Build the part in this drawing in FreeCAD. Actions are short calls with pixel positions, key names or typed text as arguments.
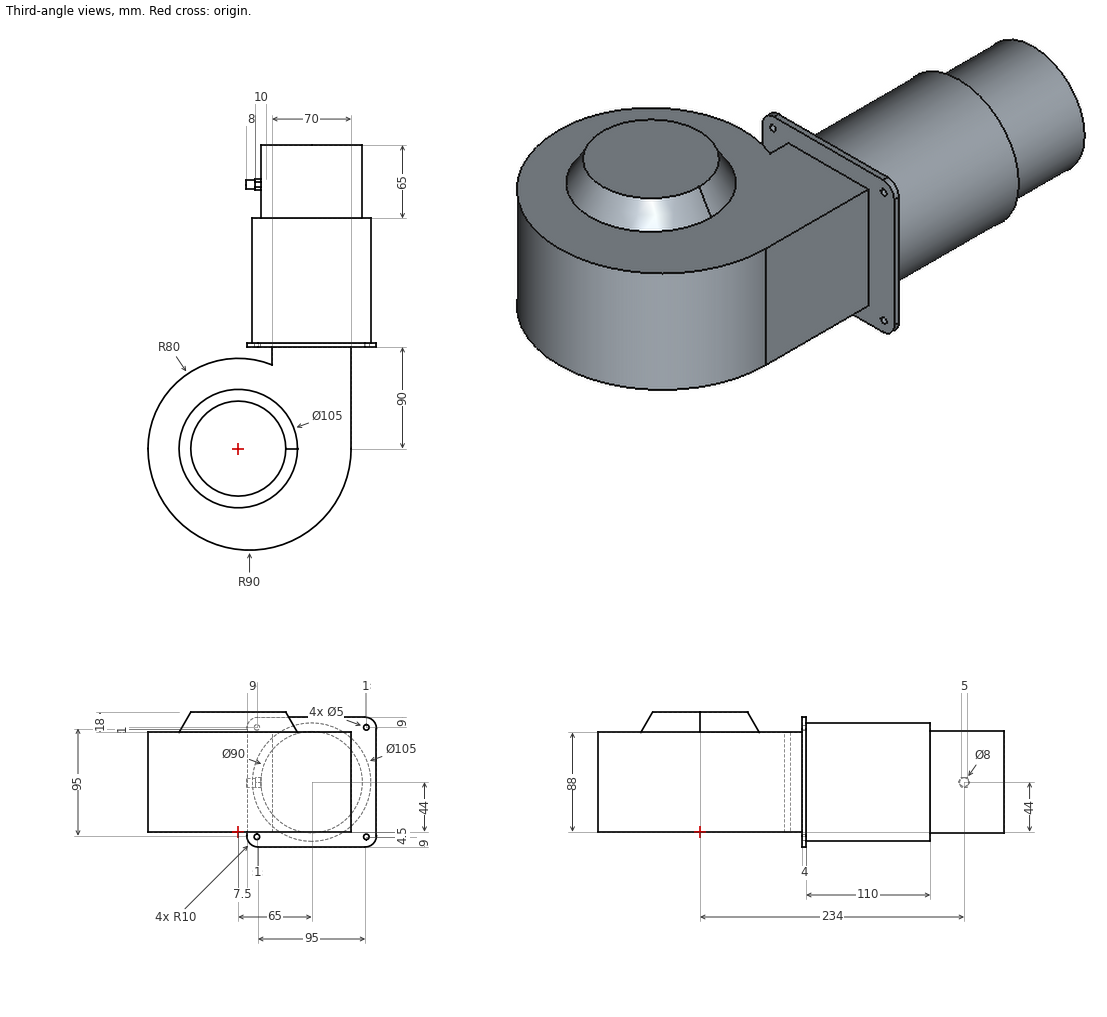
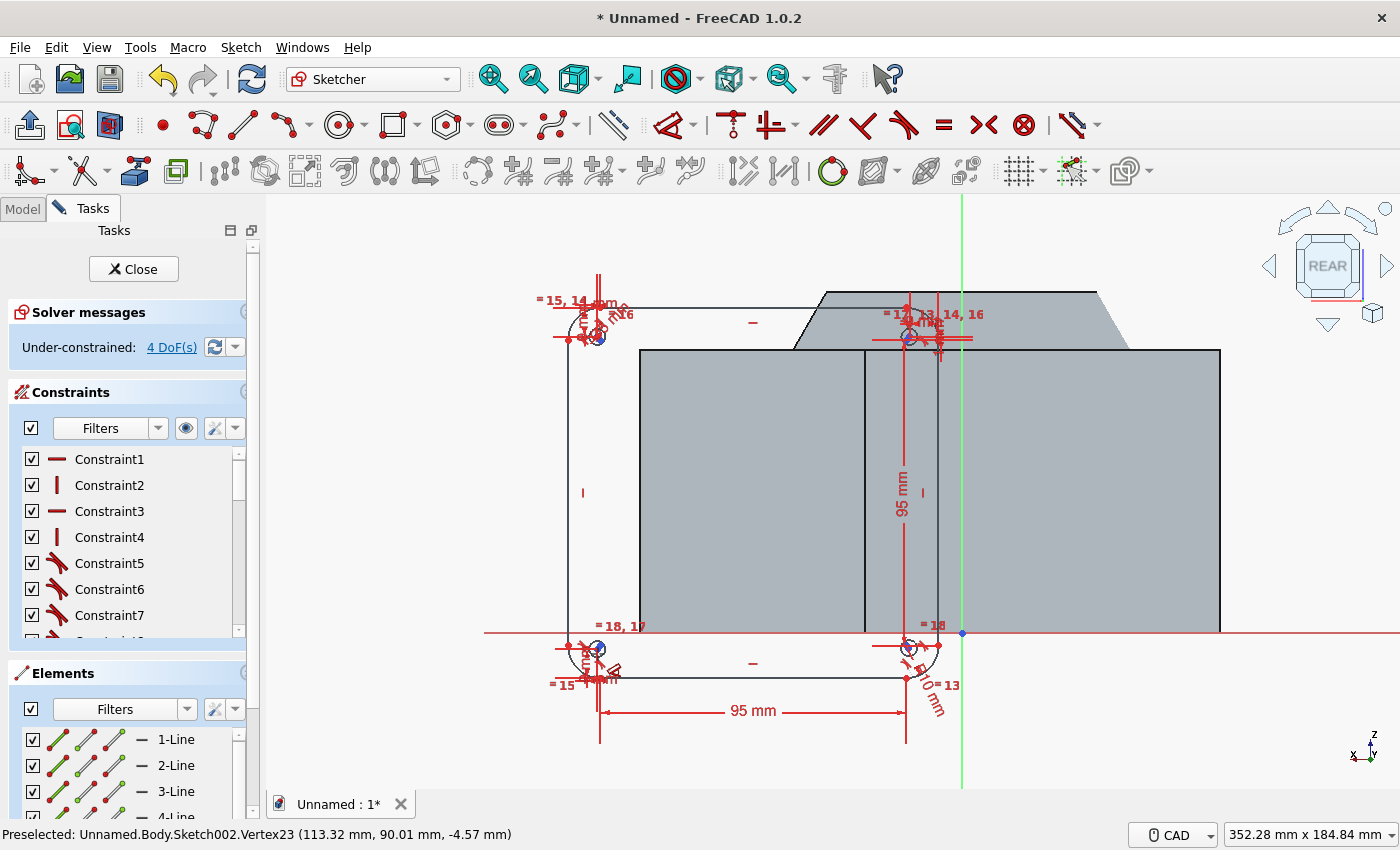
scroll(906, 678, up, 13)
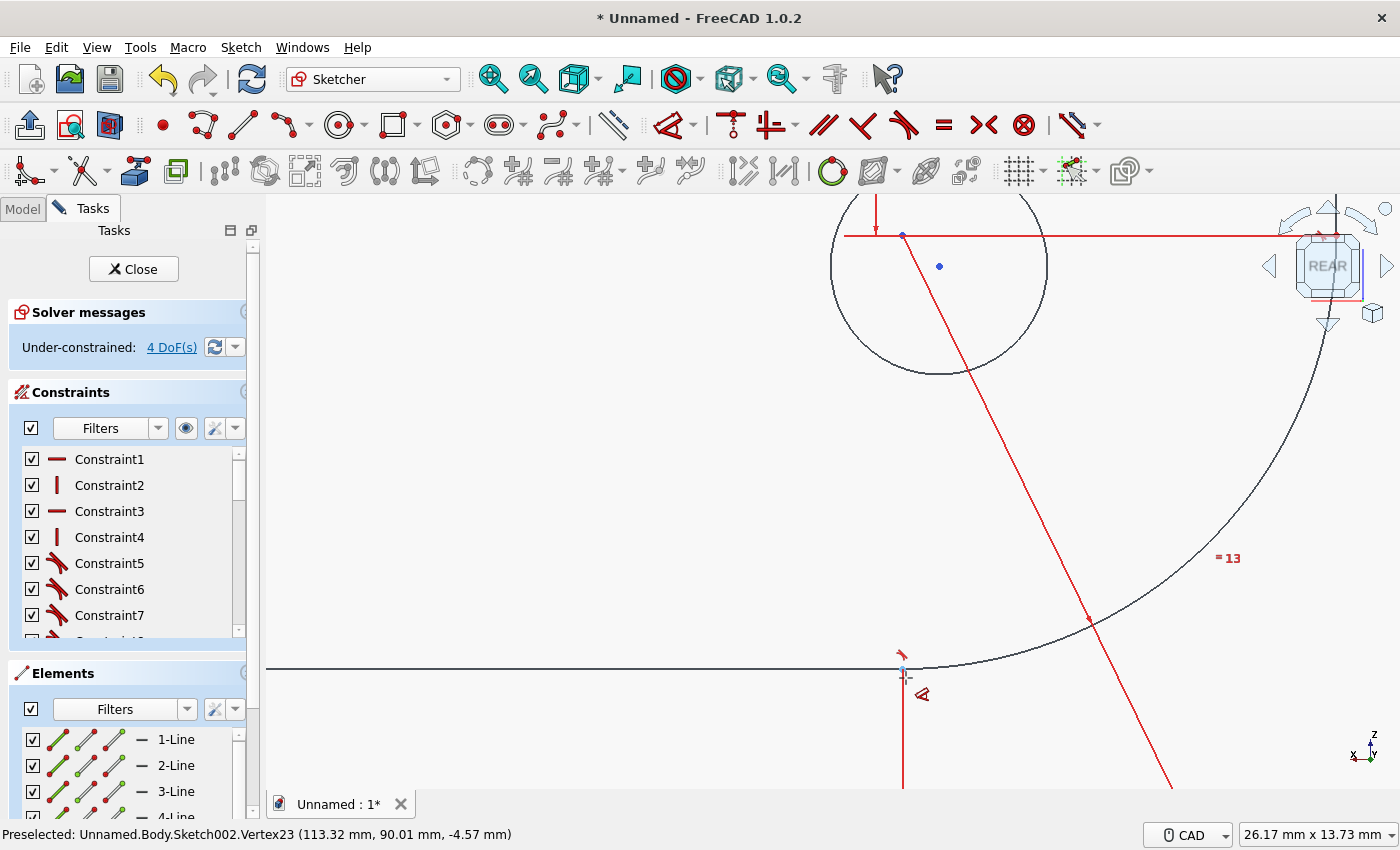
click(903, 669)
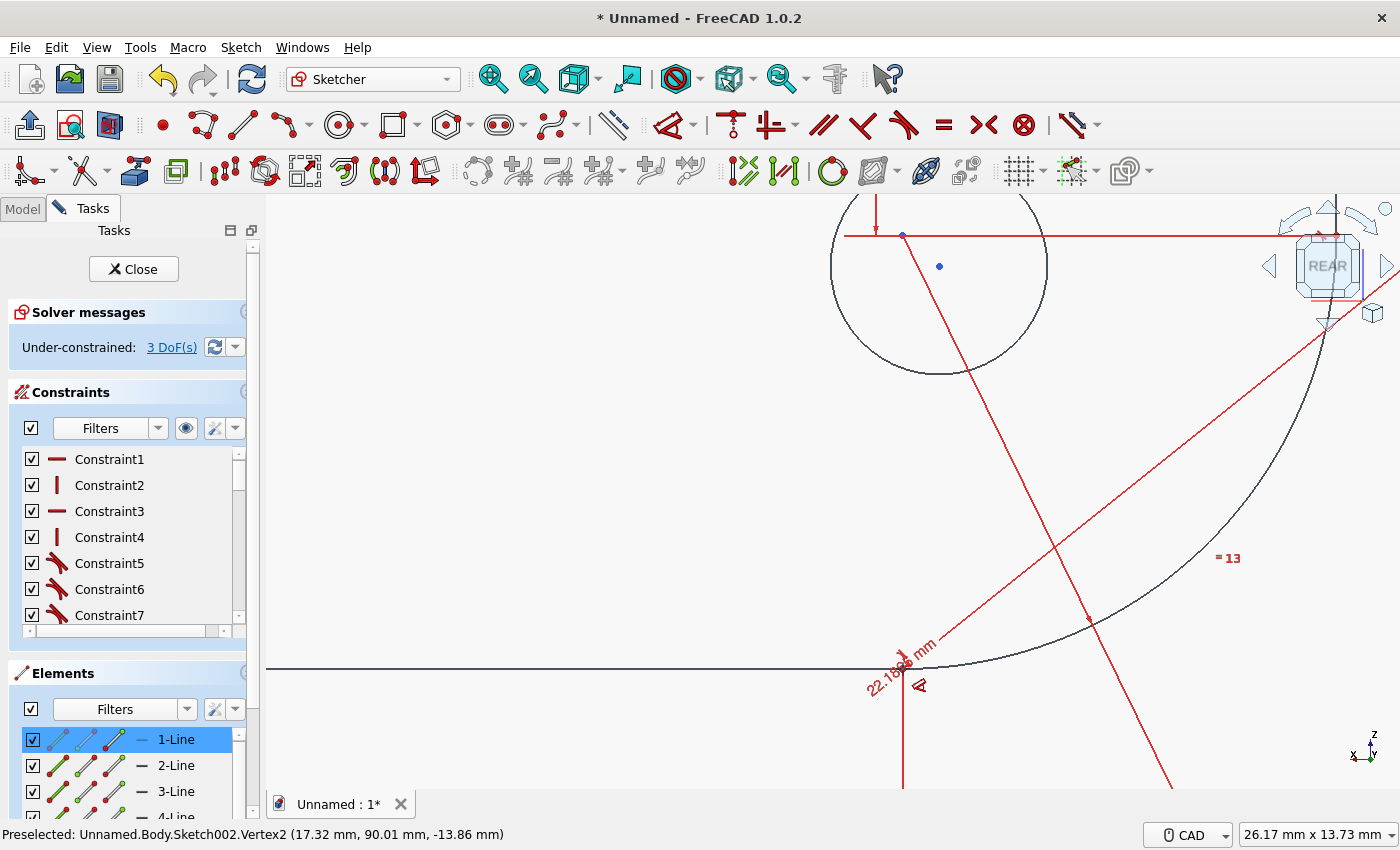
click(939, 266)
click(921, 703)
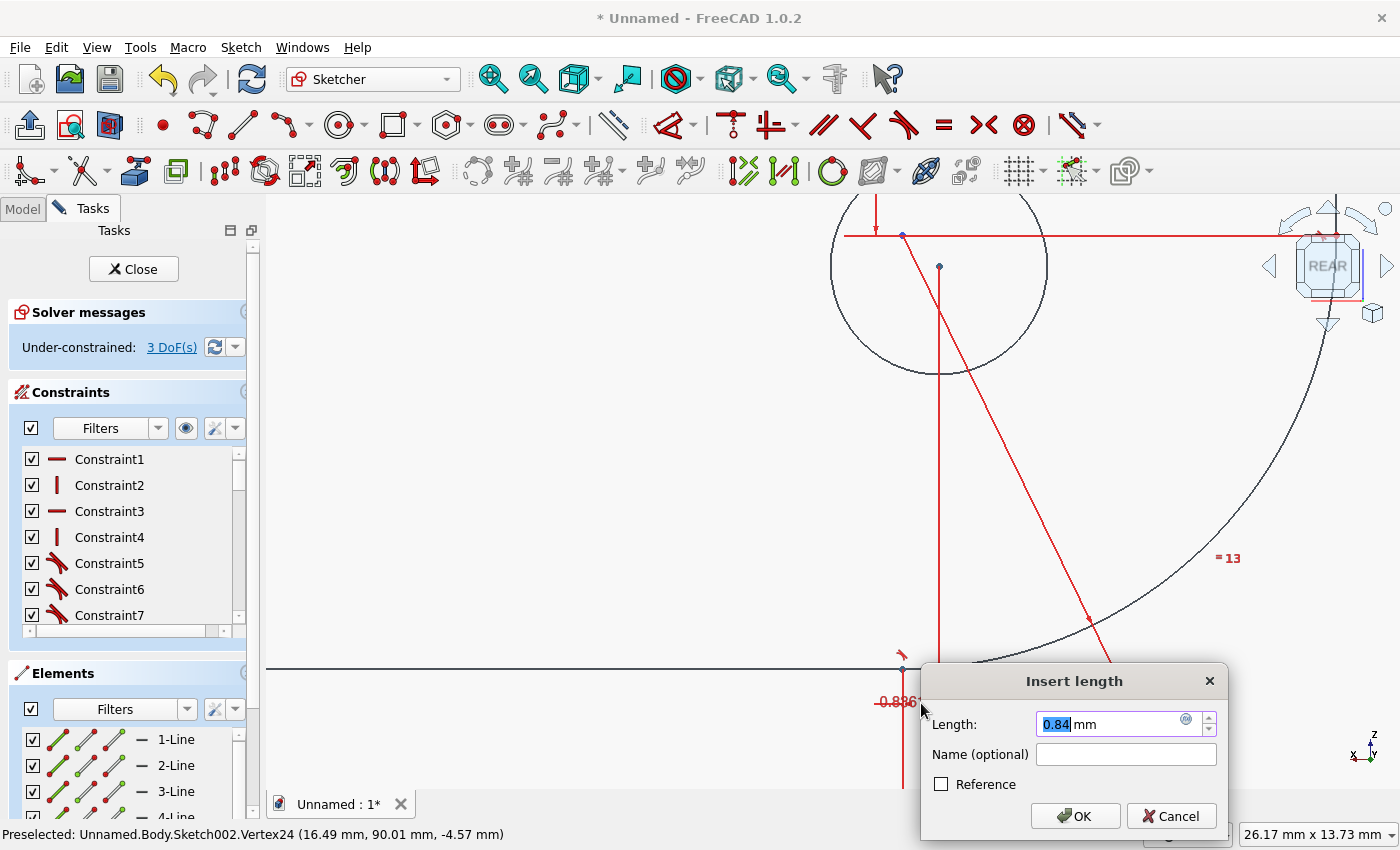
text(1)
key(Return)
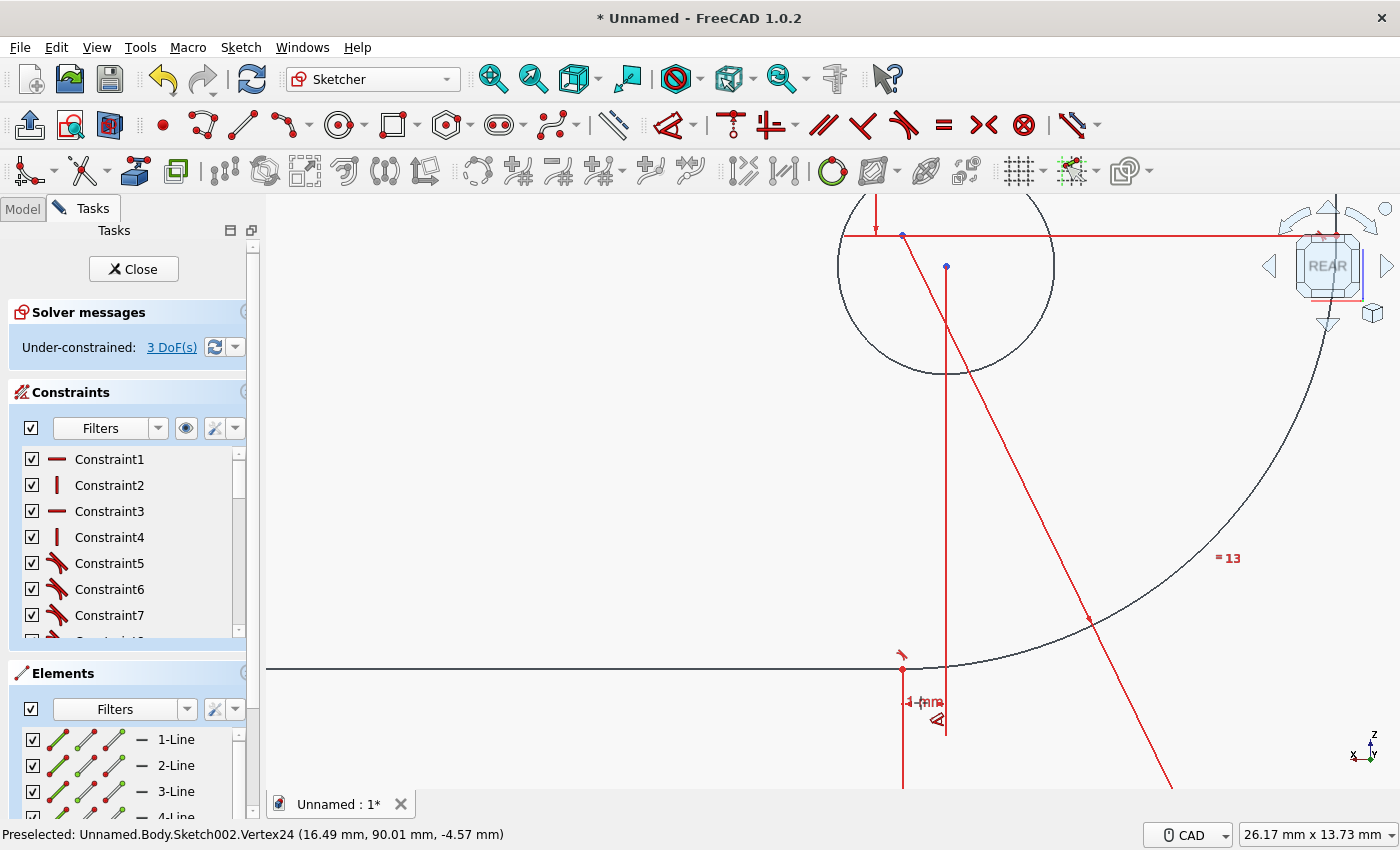
scroll(906, 678, down, 13)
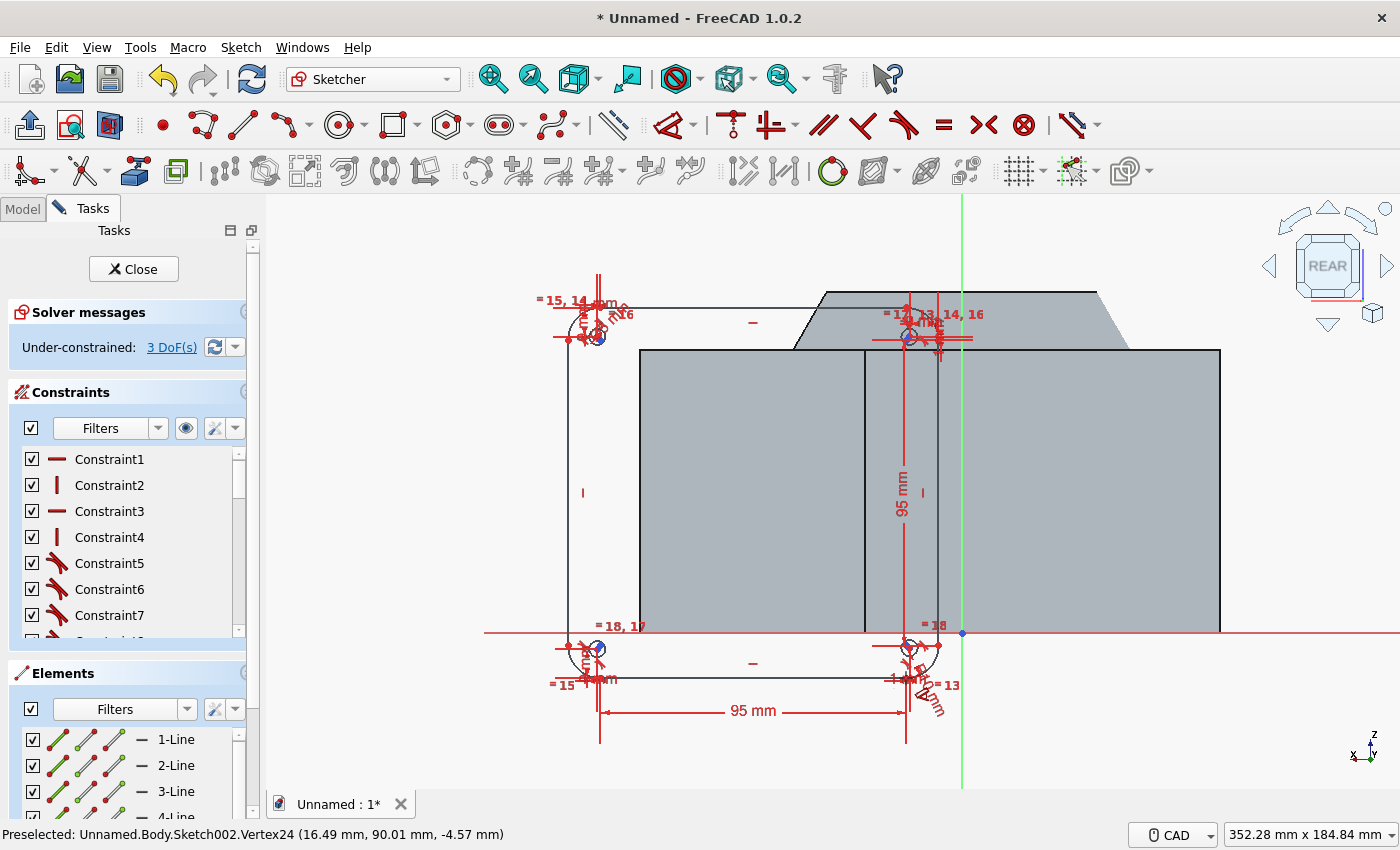
scroll(906, 678, up, 2)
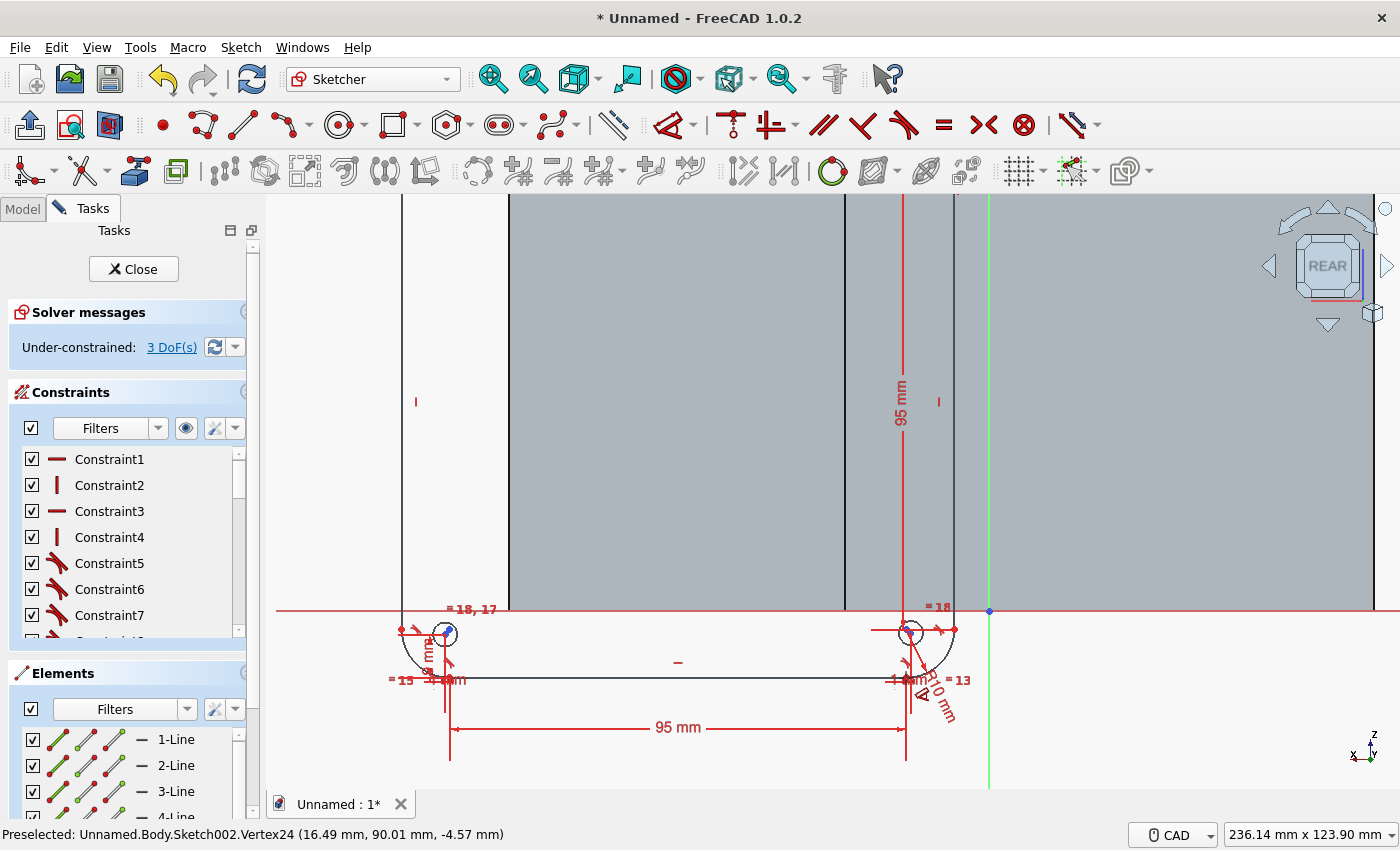
click(906, 678)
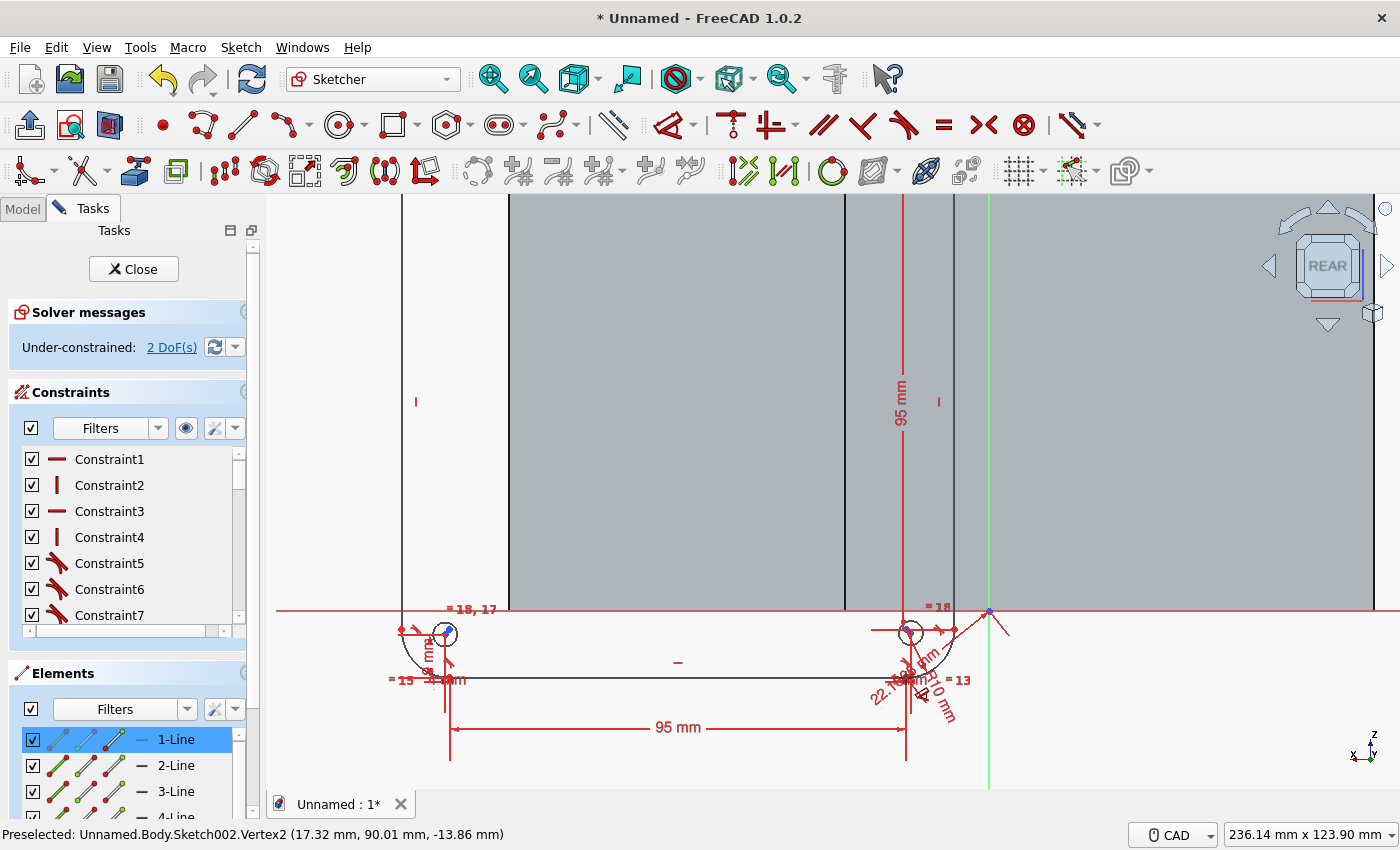
scroll(911, 633, up, 4)